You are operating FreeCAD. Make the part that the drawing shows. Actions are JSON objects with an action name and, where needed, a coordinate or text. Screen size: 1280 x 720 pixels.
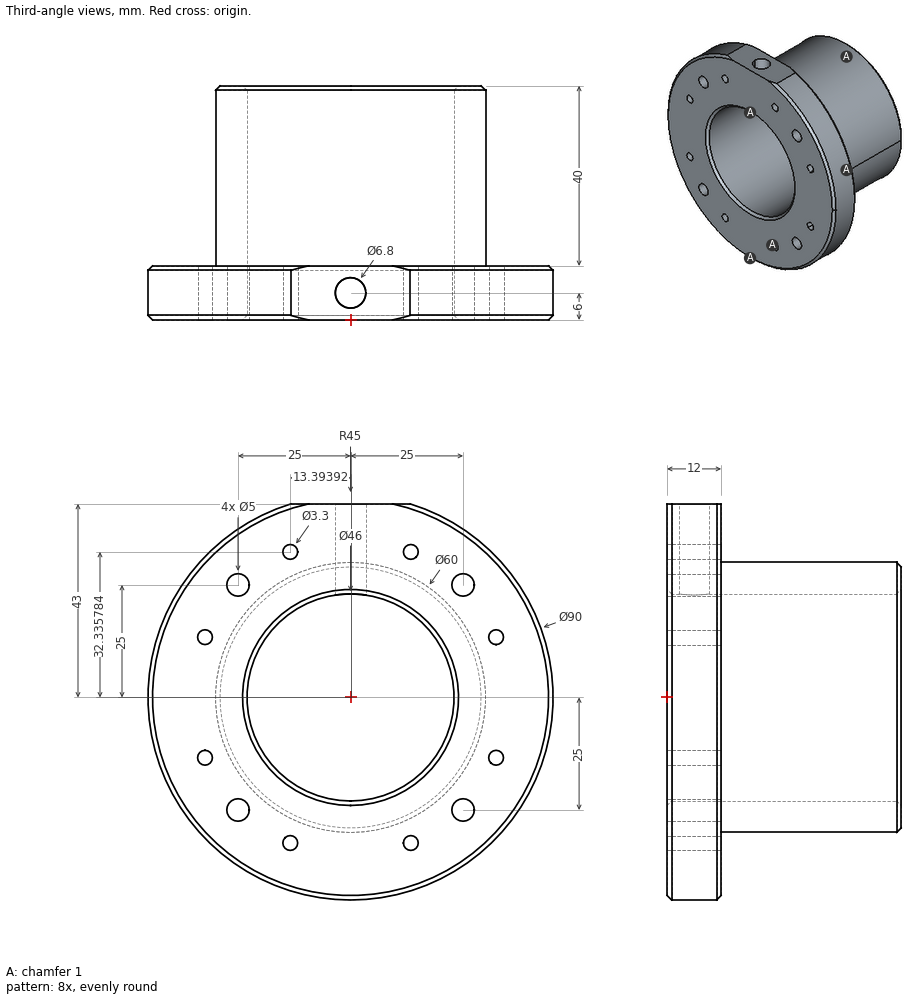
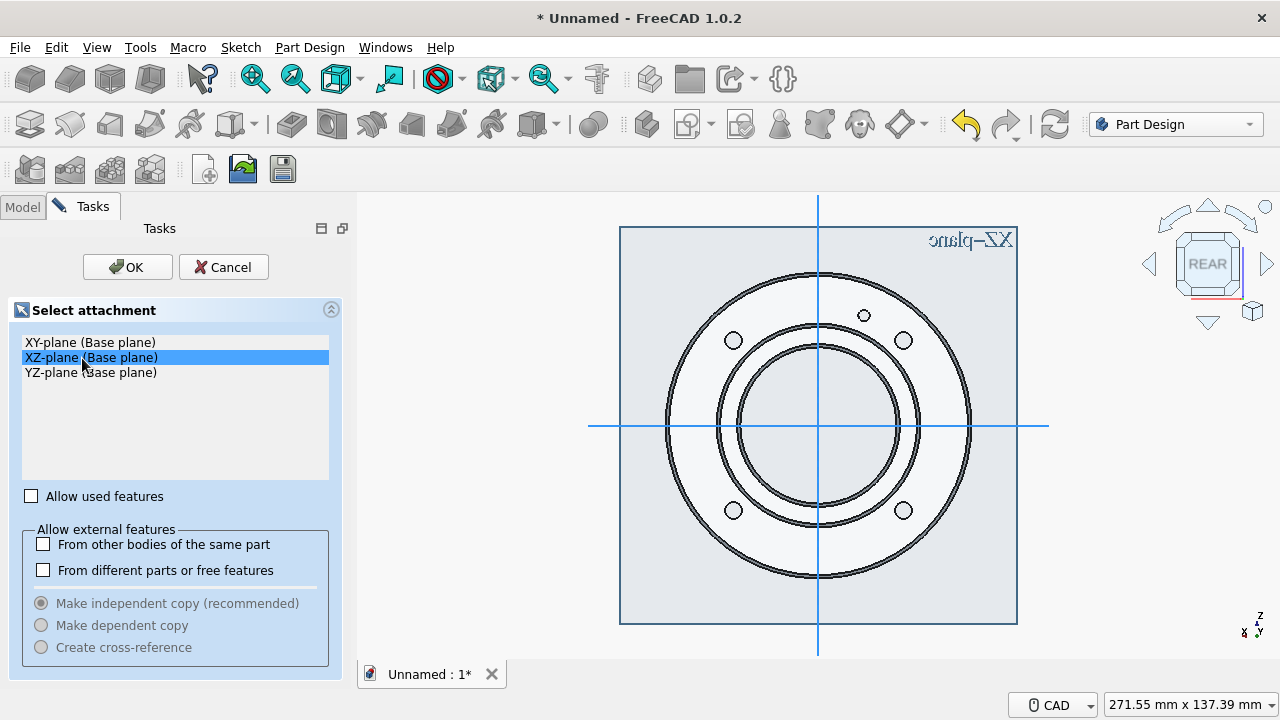
{"action": "left_click", "coordinate": [128, 267]}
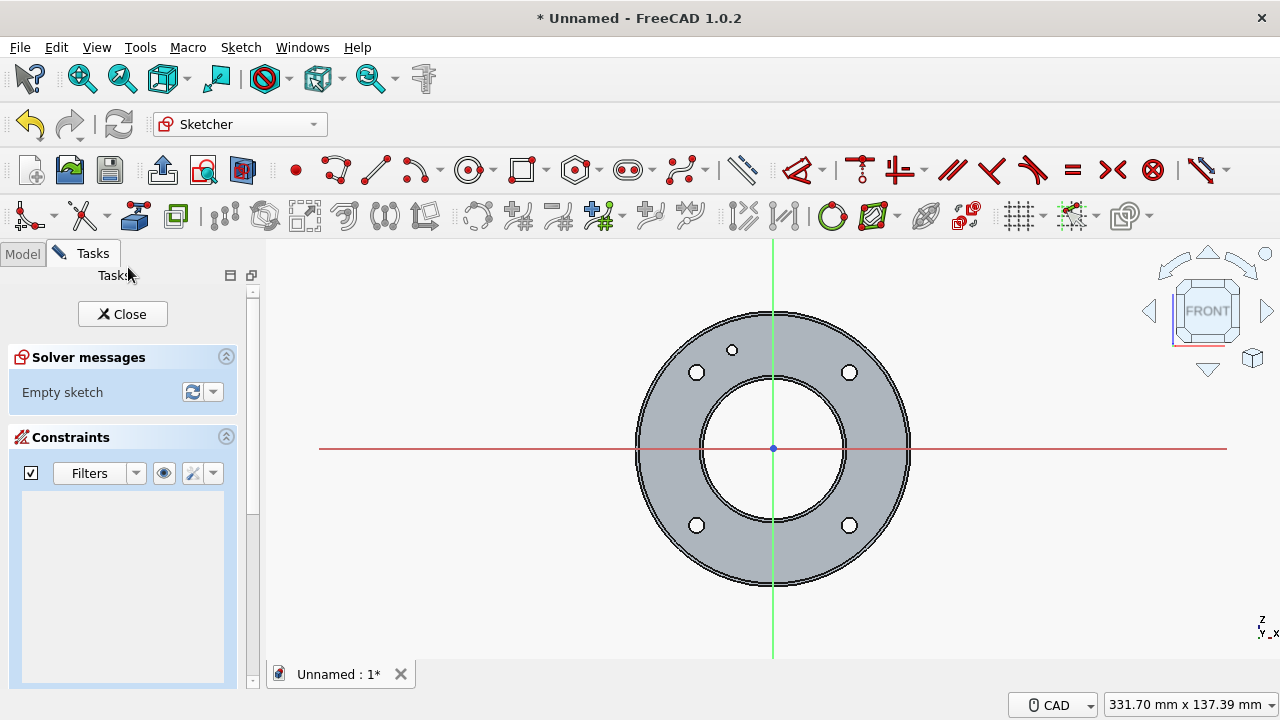
{"action": "scroll", "coordinate": [856, 297], "scroll_direction": "up", "scroll_amount": 3}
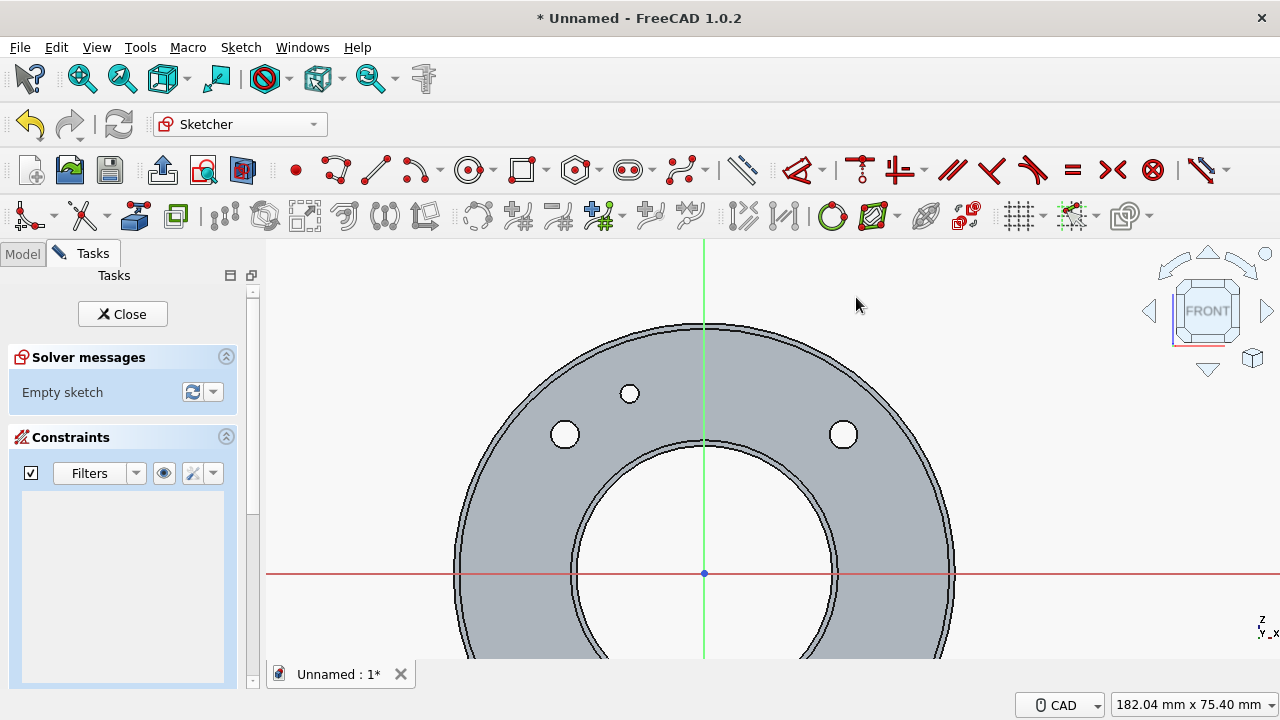
{"action": "left_click", "coordinate": [376, 170]}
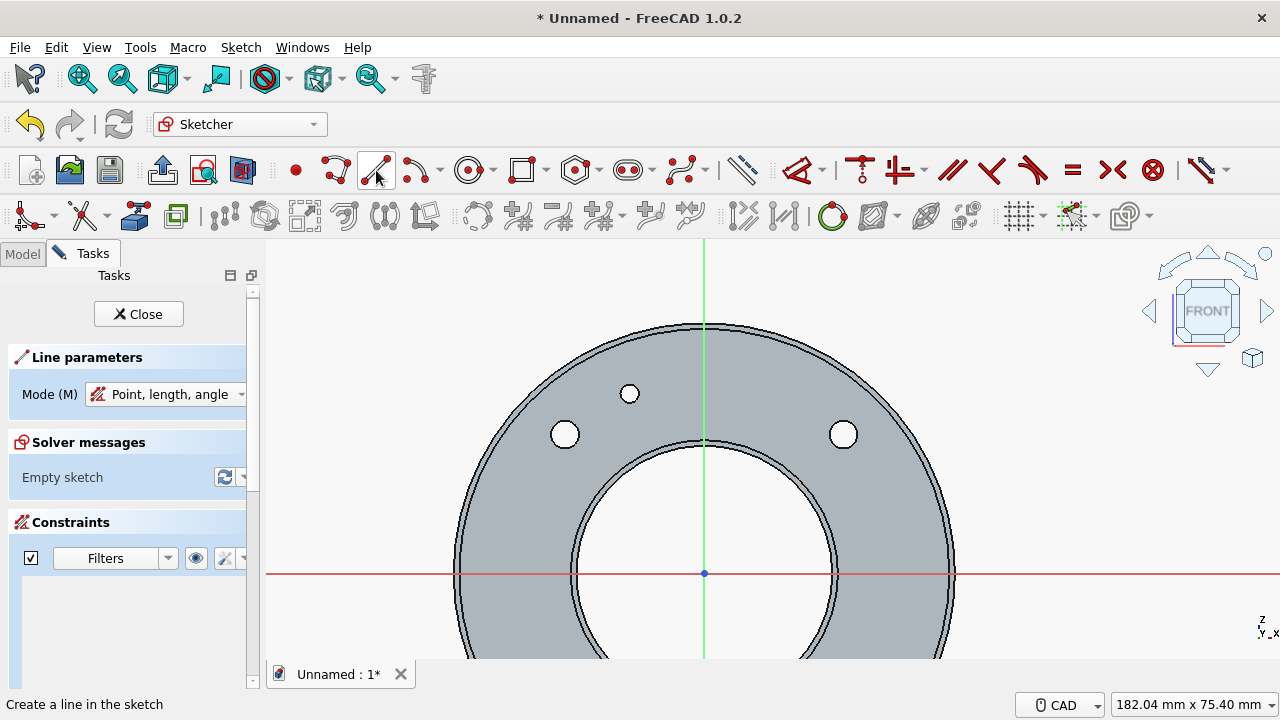
{"action": "left_click", "coordinate": [630, 334]}
{"action": "left_click", "coordinate": [778, 334]}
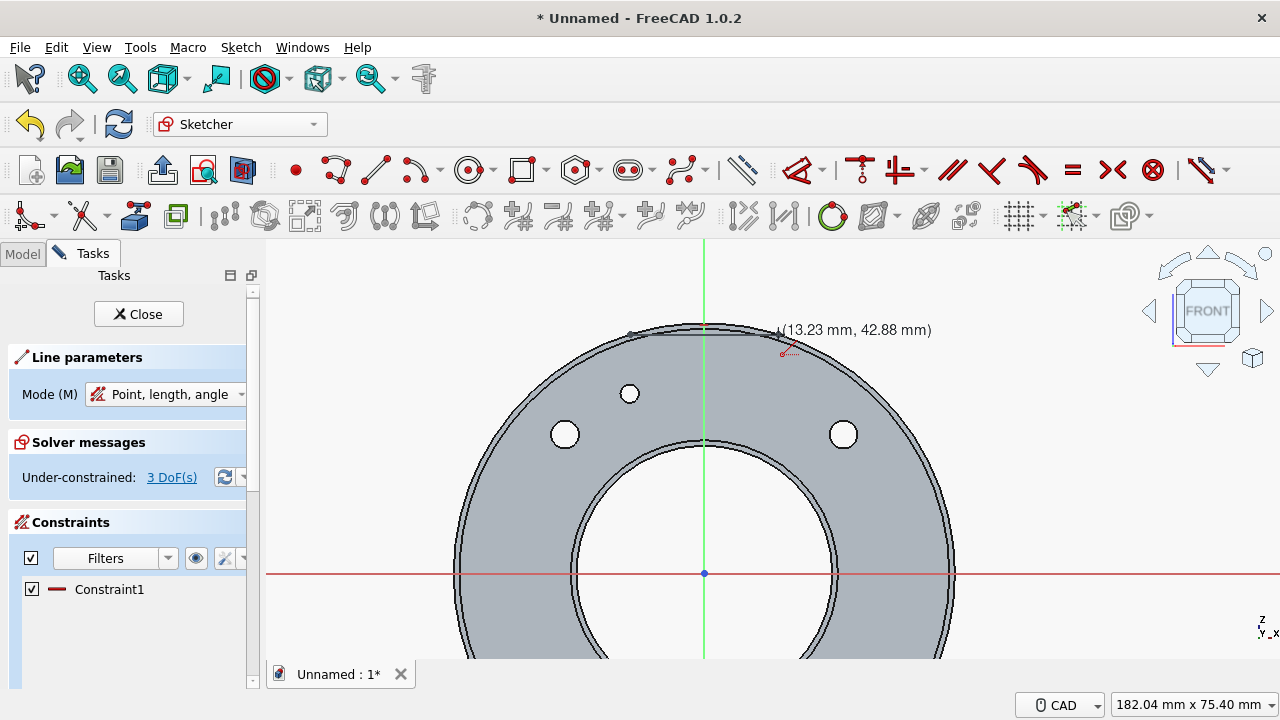
{"action": "key", "text": "g 3 a"}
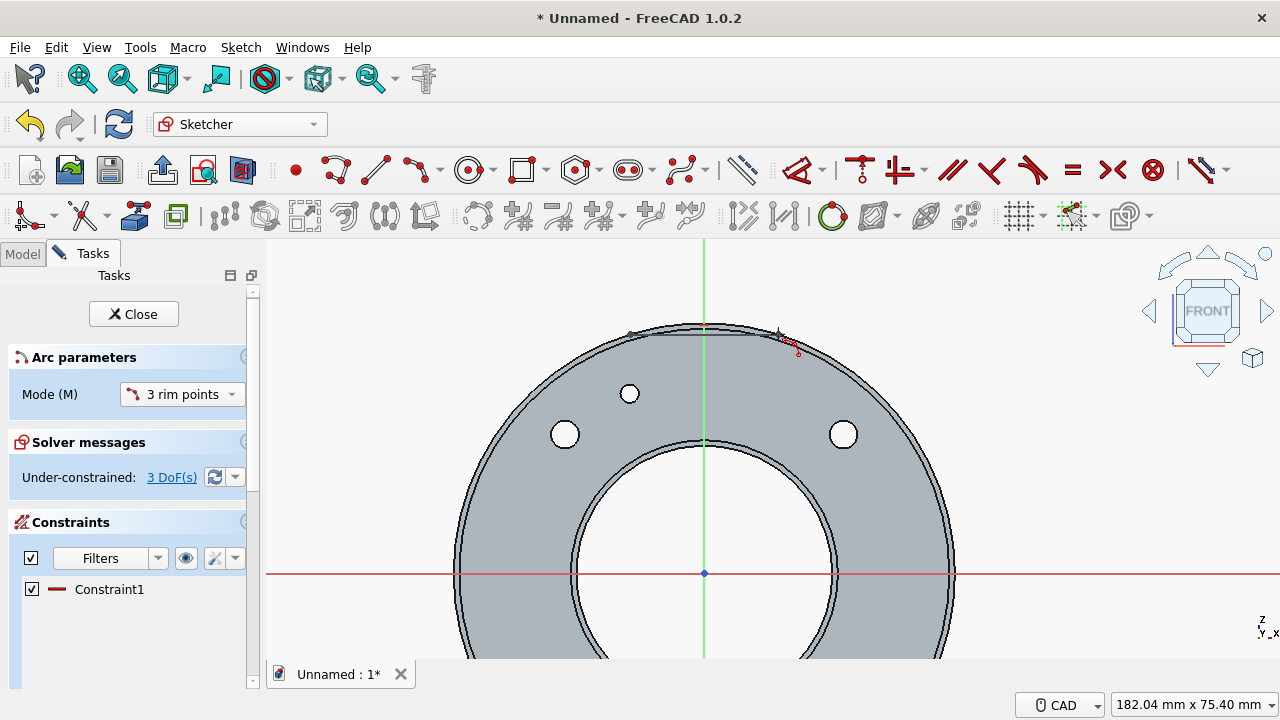
{"action": "left_click", "coordinate": [778, 335]}
{"action": "left_click", "coordinate": [630, 335]}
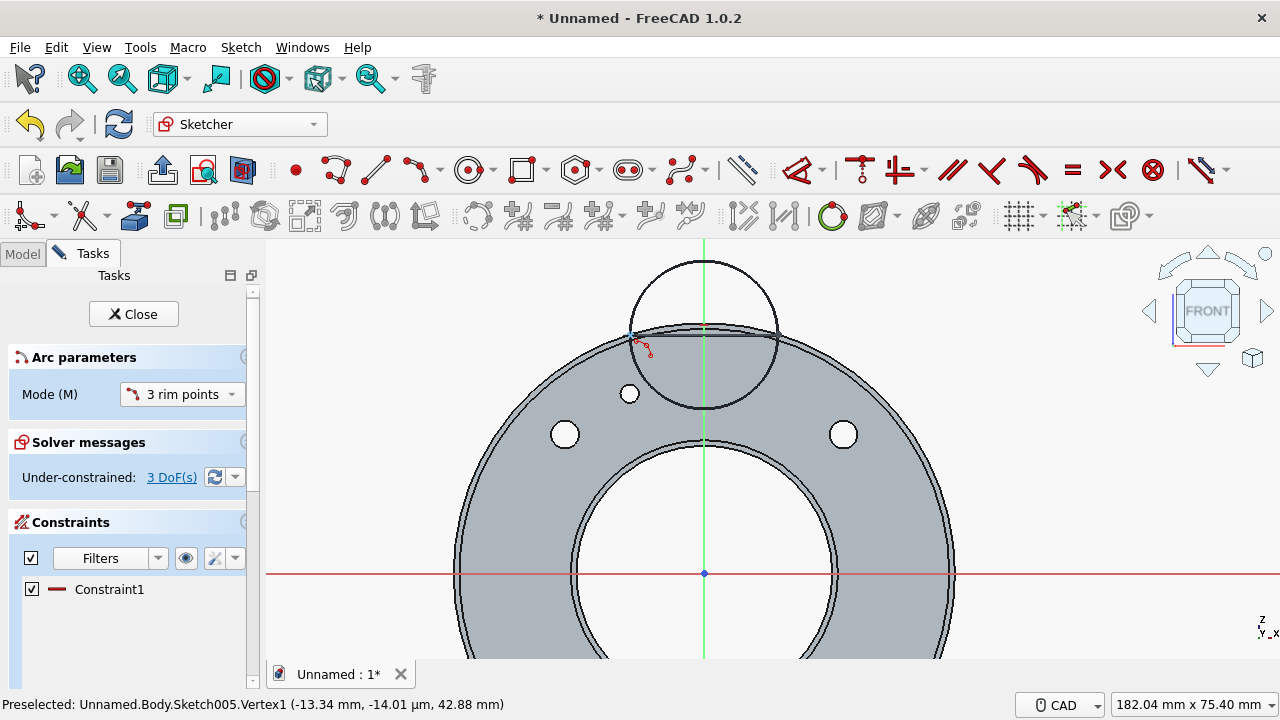
{"action": "scroll", "coordinate": [719, 324], "scroll_direction": "up", "scroll_amount": 2}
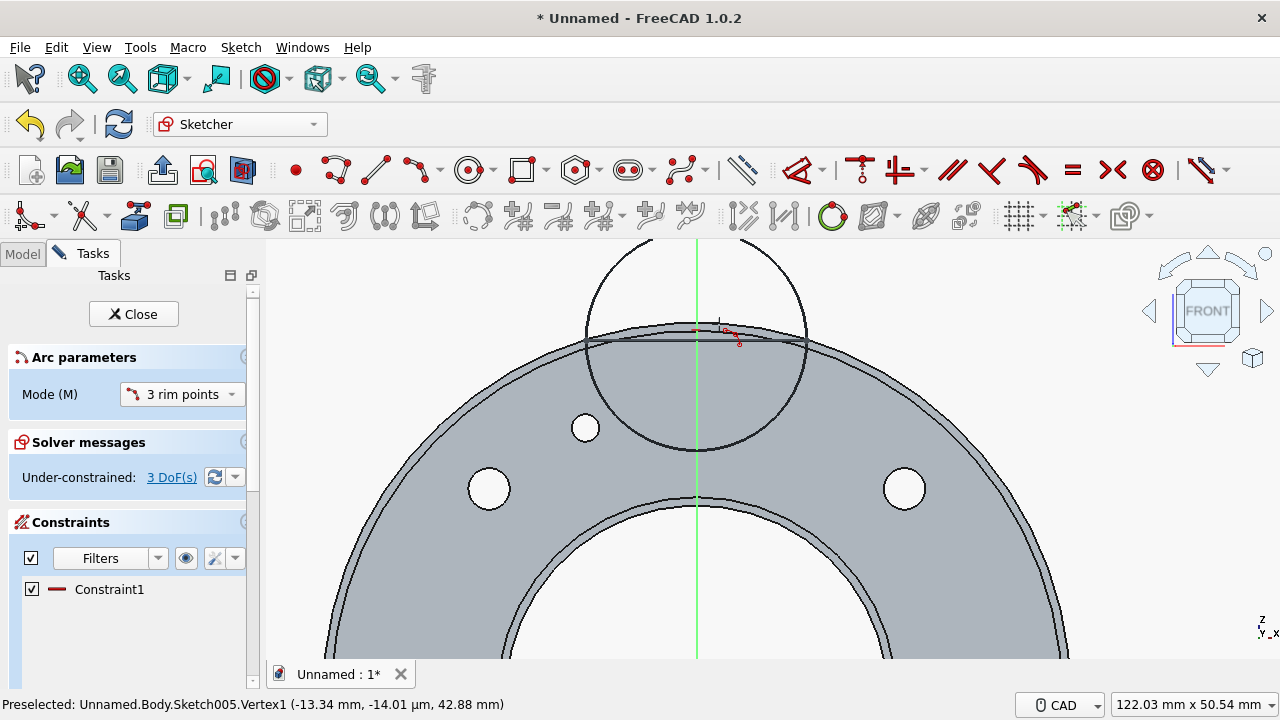
{"action": "left_click", "coordinate": [719, 323]}
{"action": "key", "text": "Escape"}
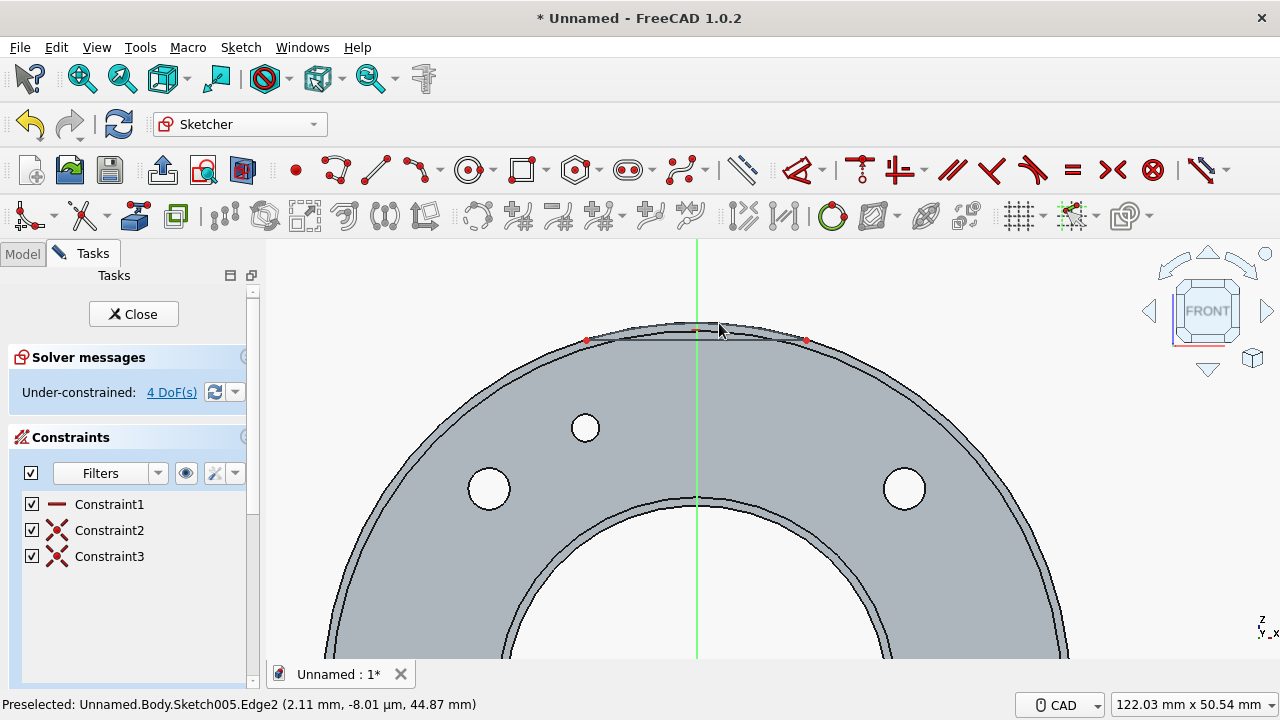
{"action": "scroll", "coordinate": [720, 326], "scroll_direction": "down", "scroll_amount": 2}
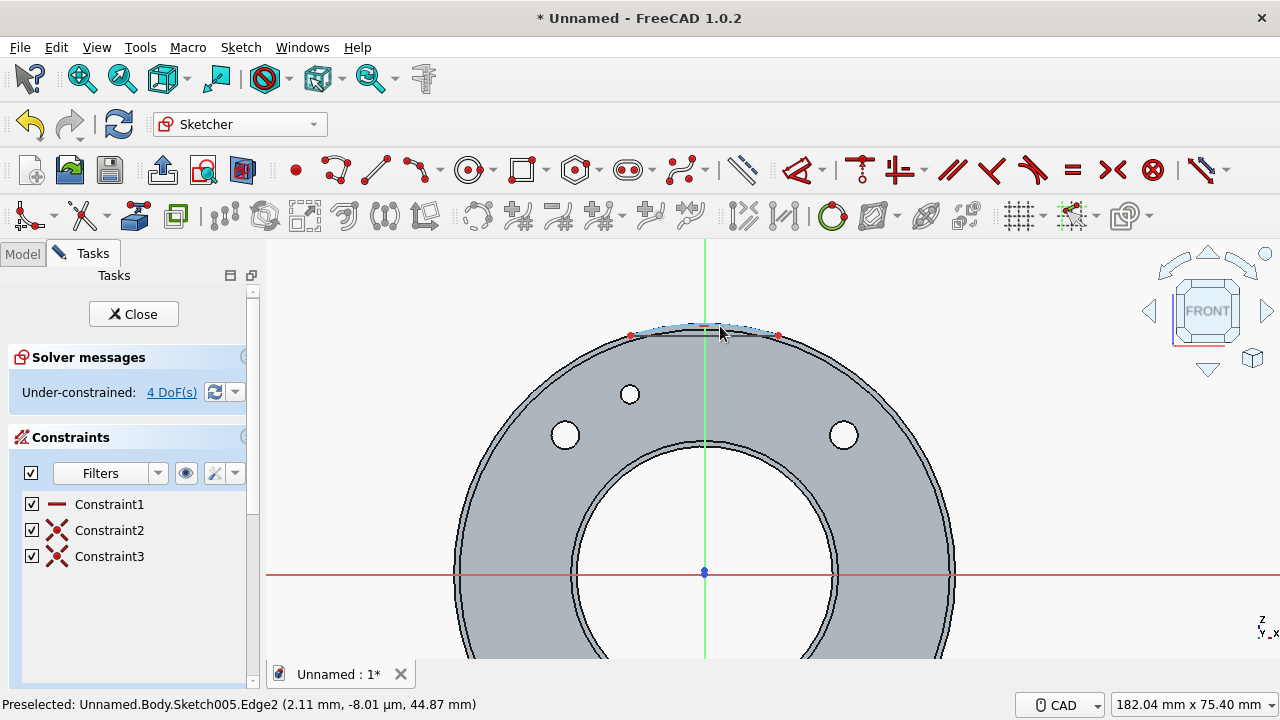
{"action": "left_click_drag", "start_coordinate": [694, 560], "coordinate": [715, 585]}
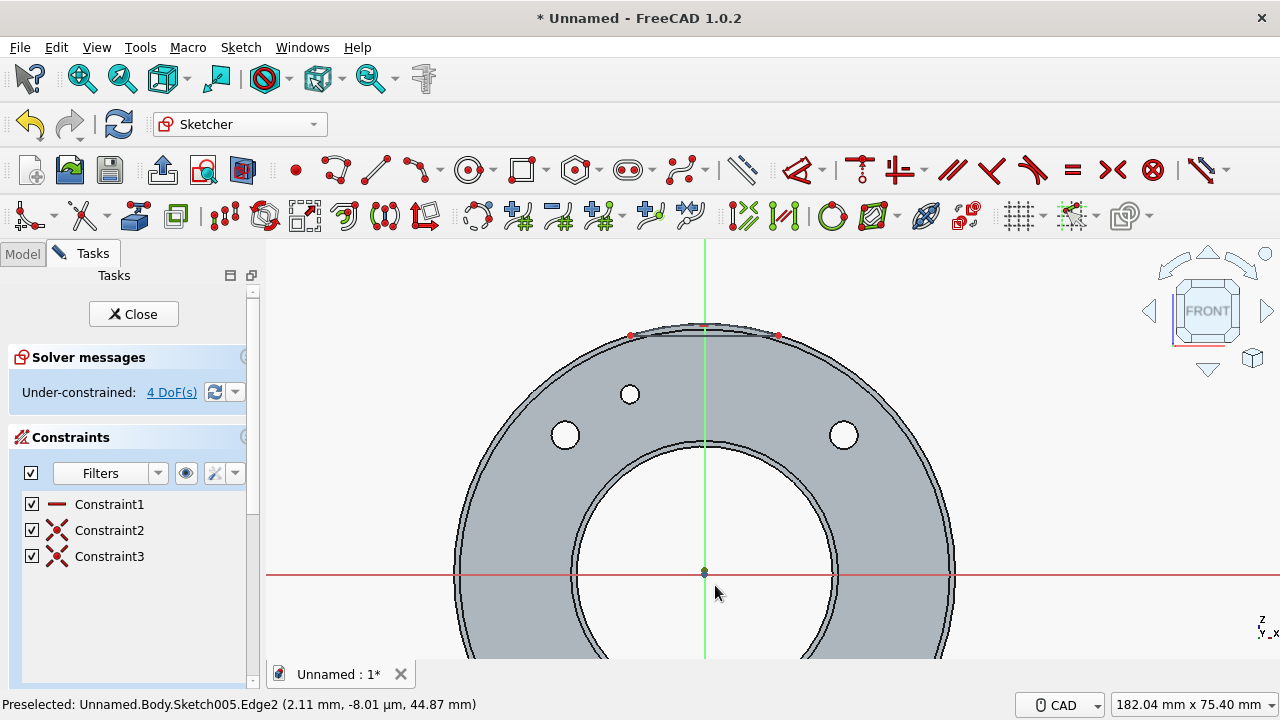
{"action": "key", "text": "c"}